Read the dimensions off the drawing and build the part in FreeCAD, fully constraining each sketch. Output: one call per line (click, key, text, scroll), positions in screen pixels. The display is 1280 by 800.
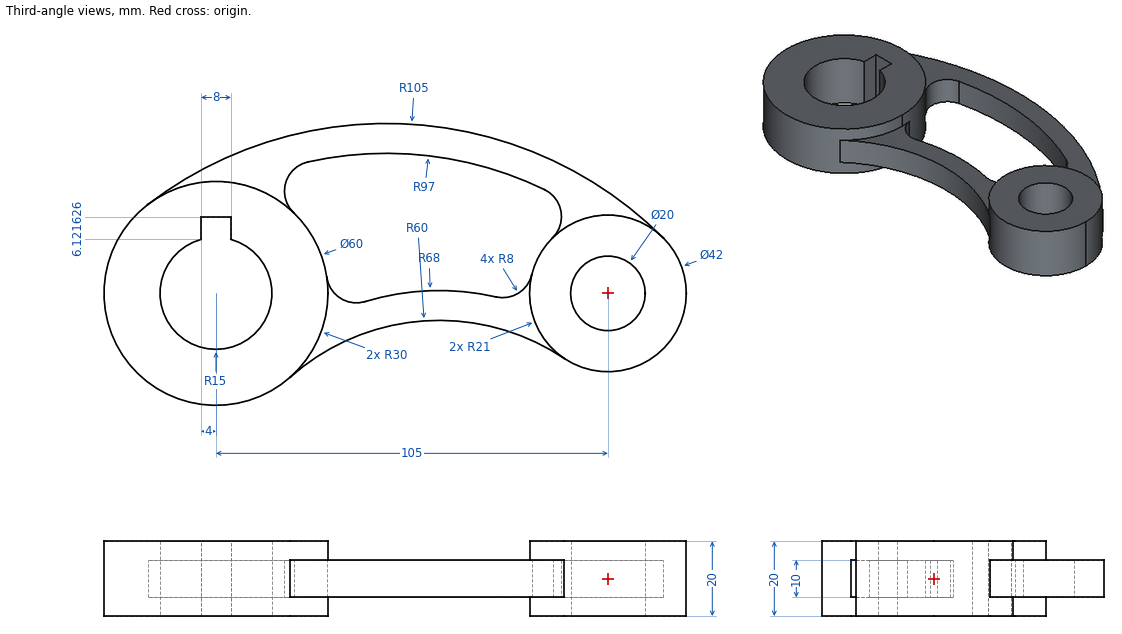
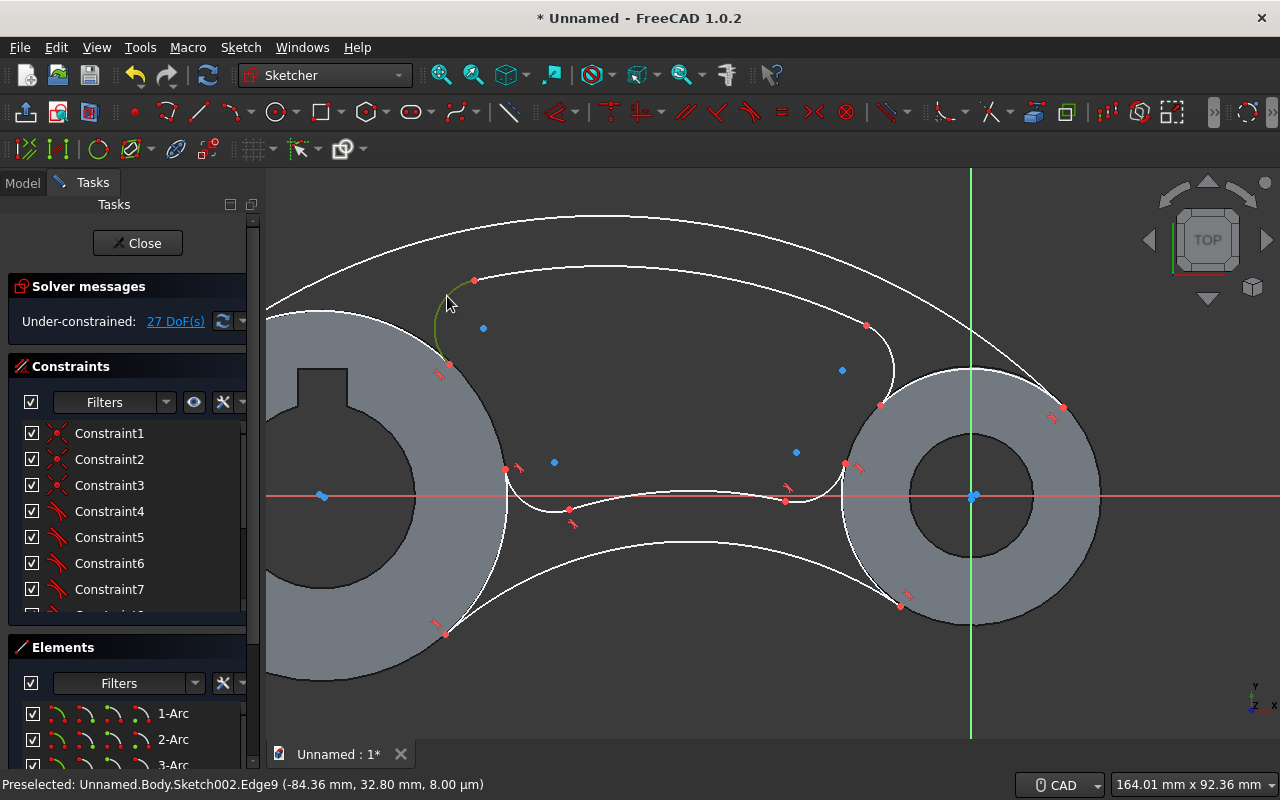
click(753, 284)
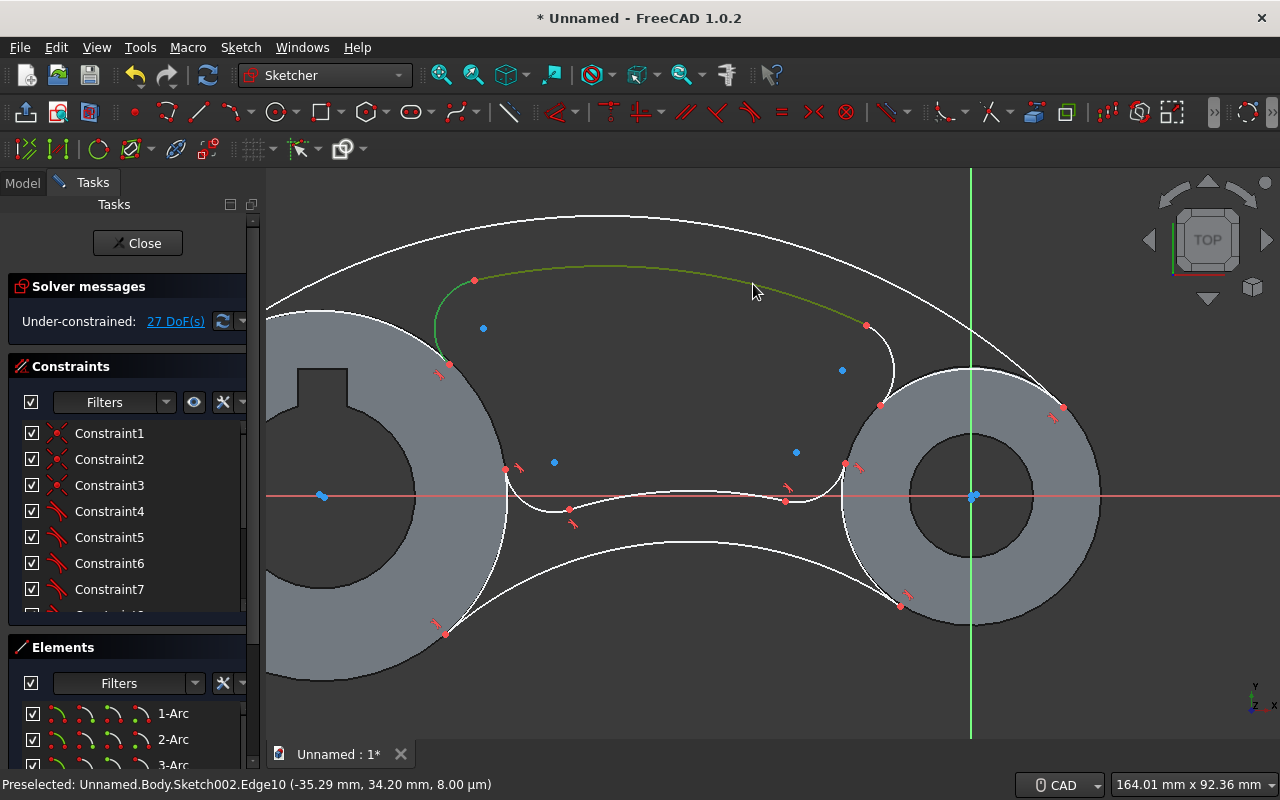
key(t)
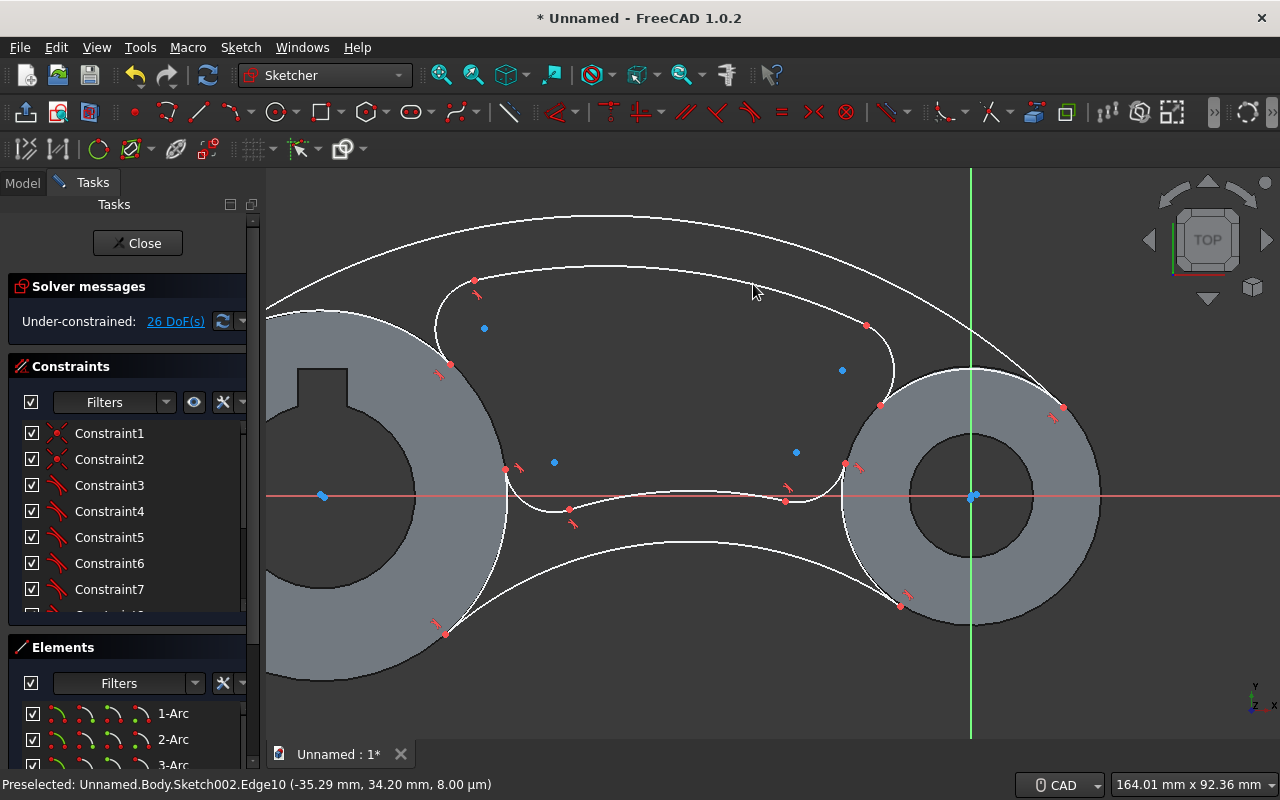
click(753, 284)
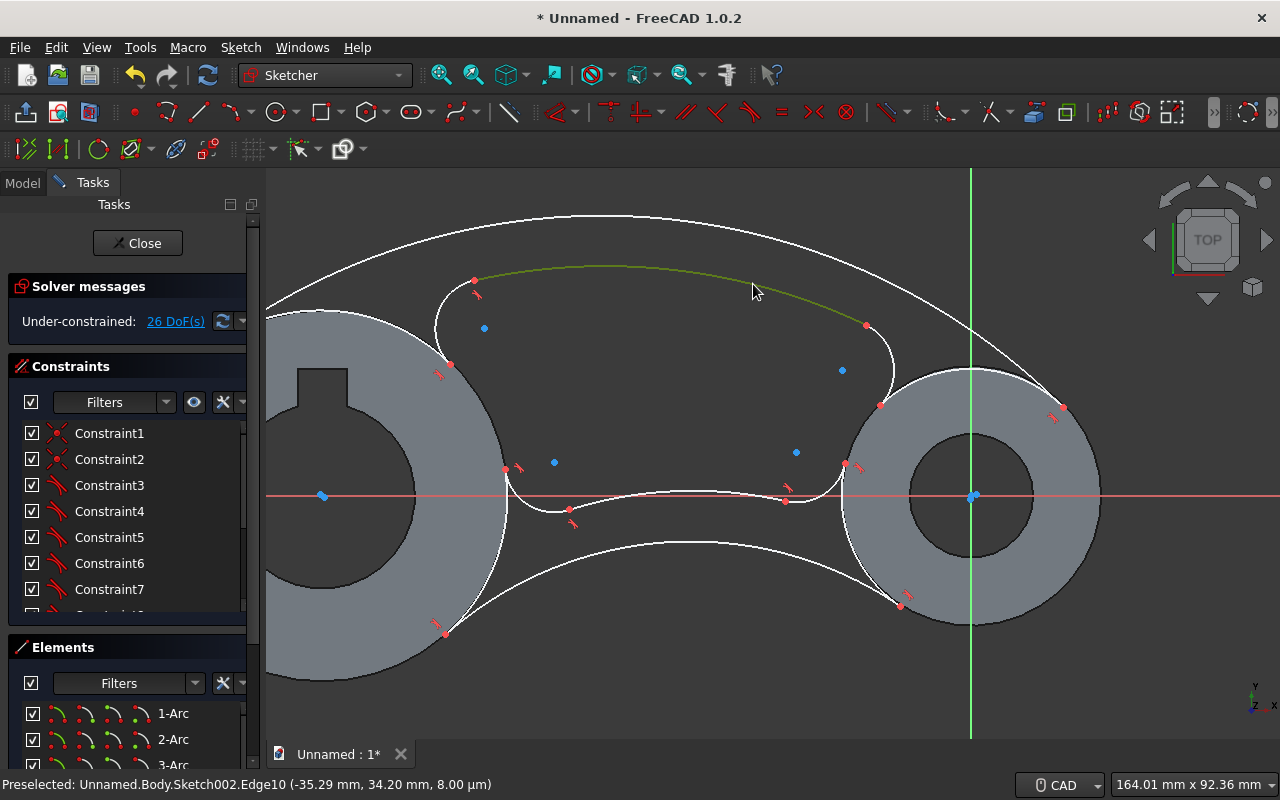
scroll(893, 381, up, 2)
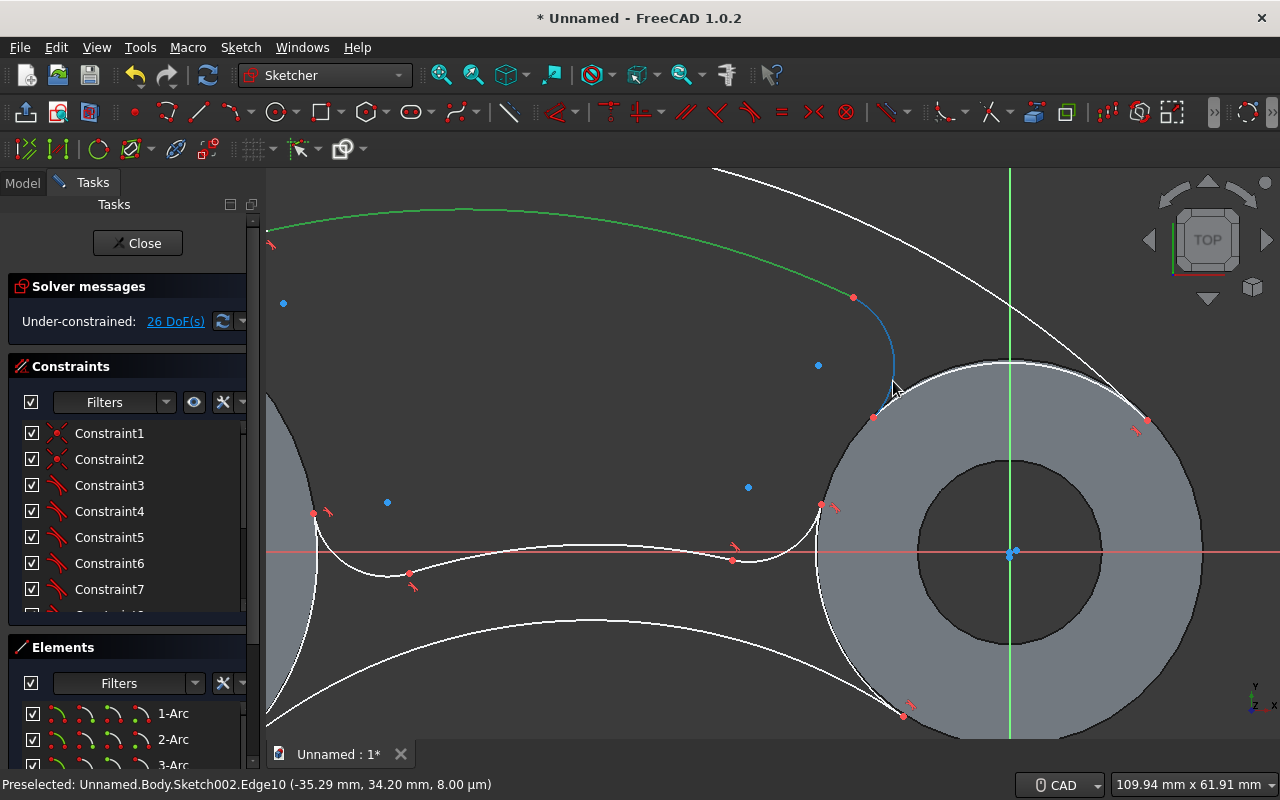
click(893, 381)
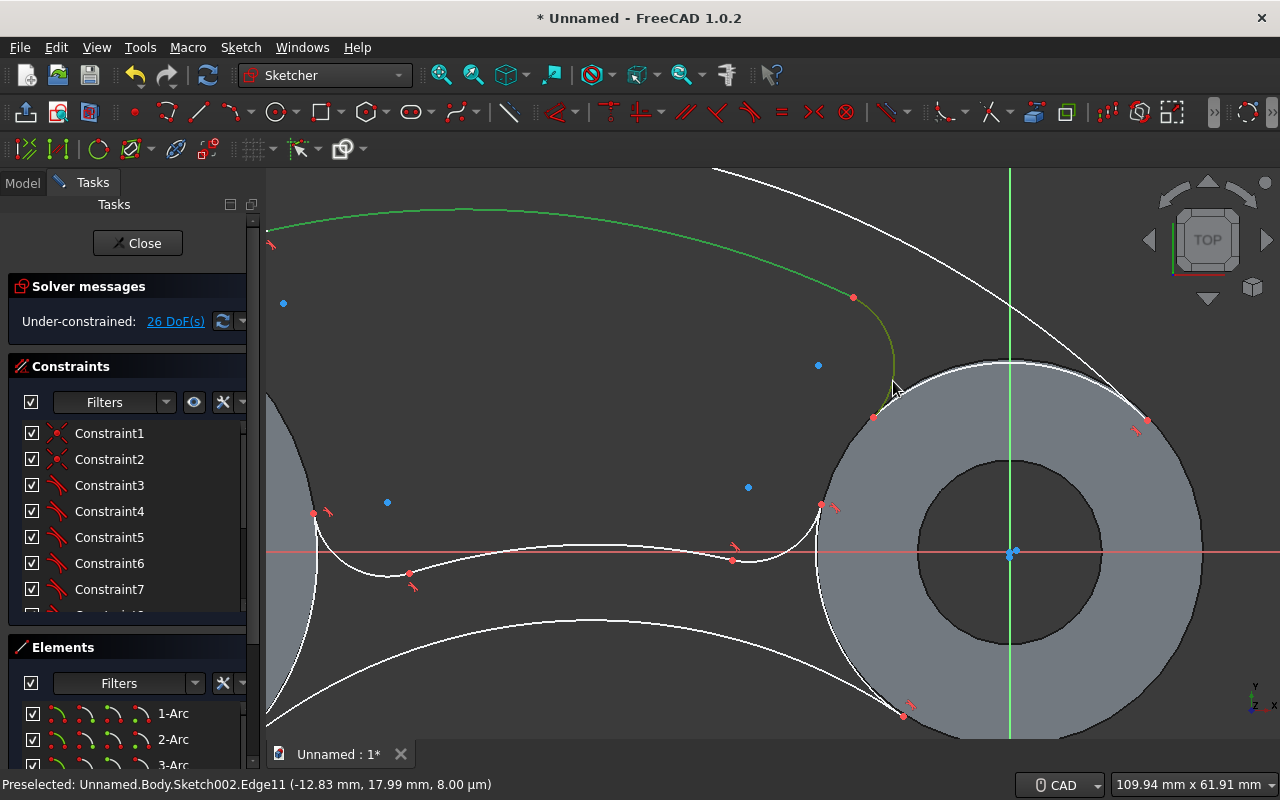
key(t)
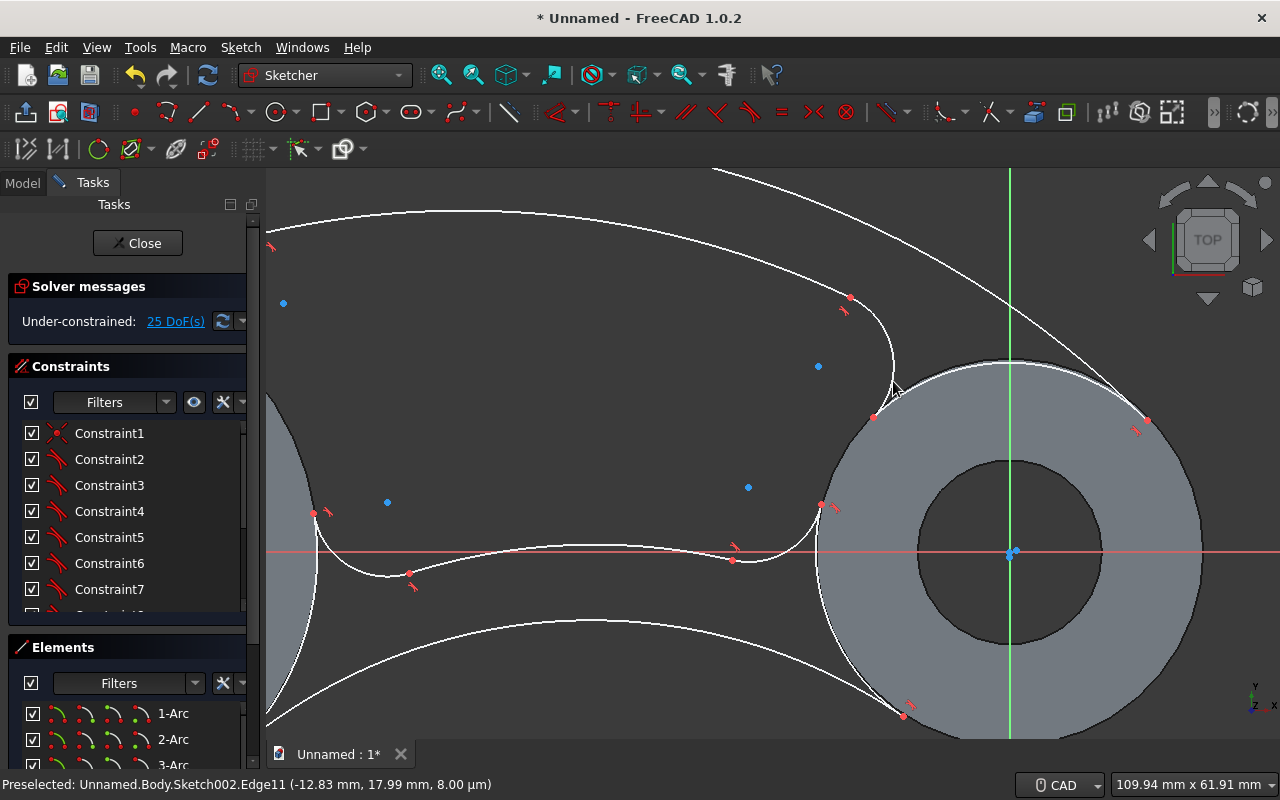
click(892, 380)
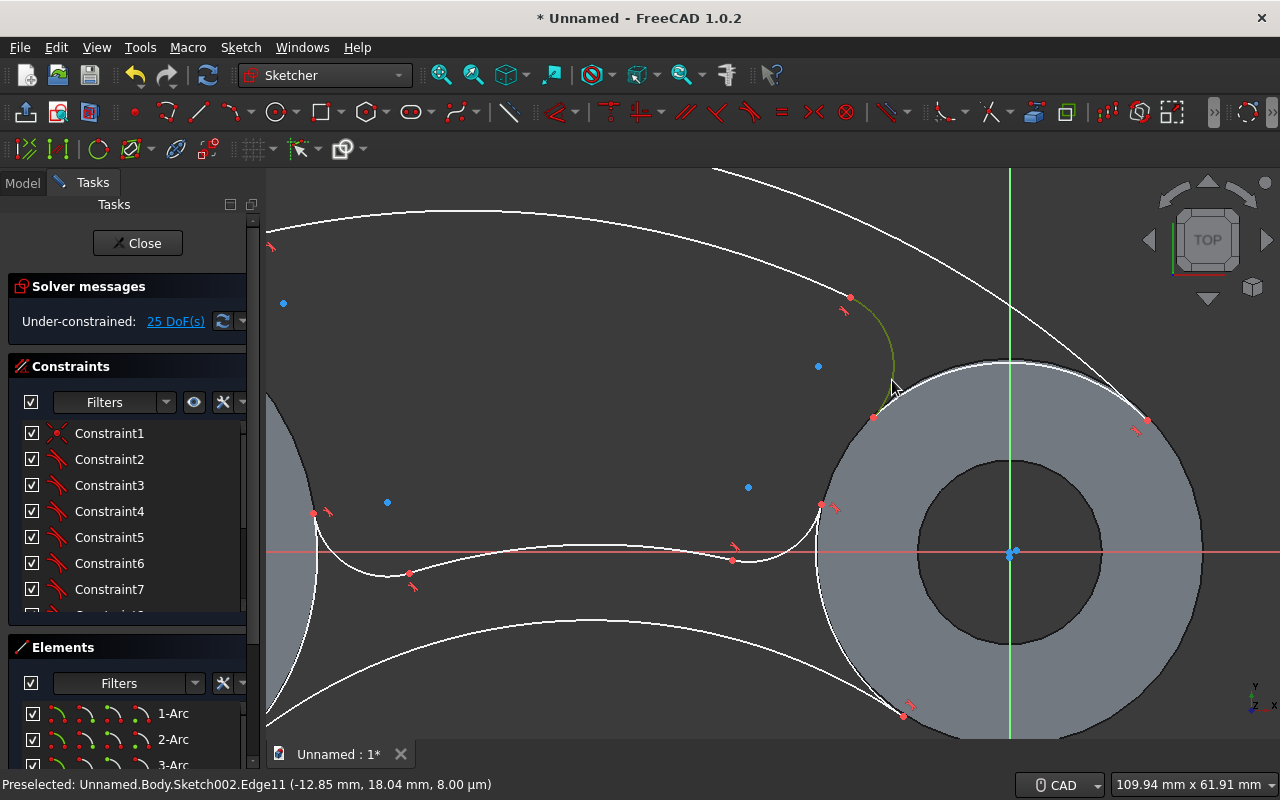
click(1070, 373)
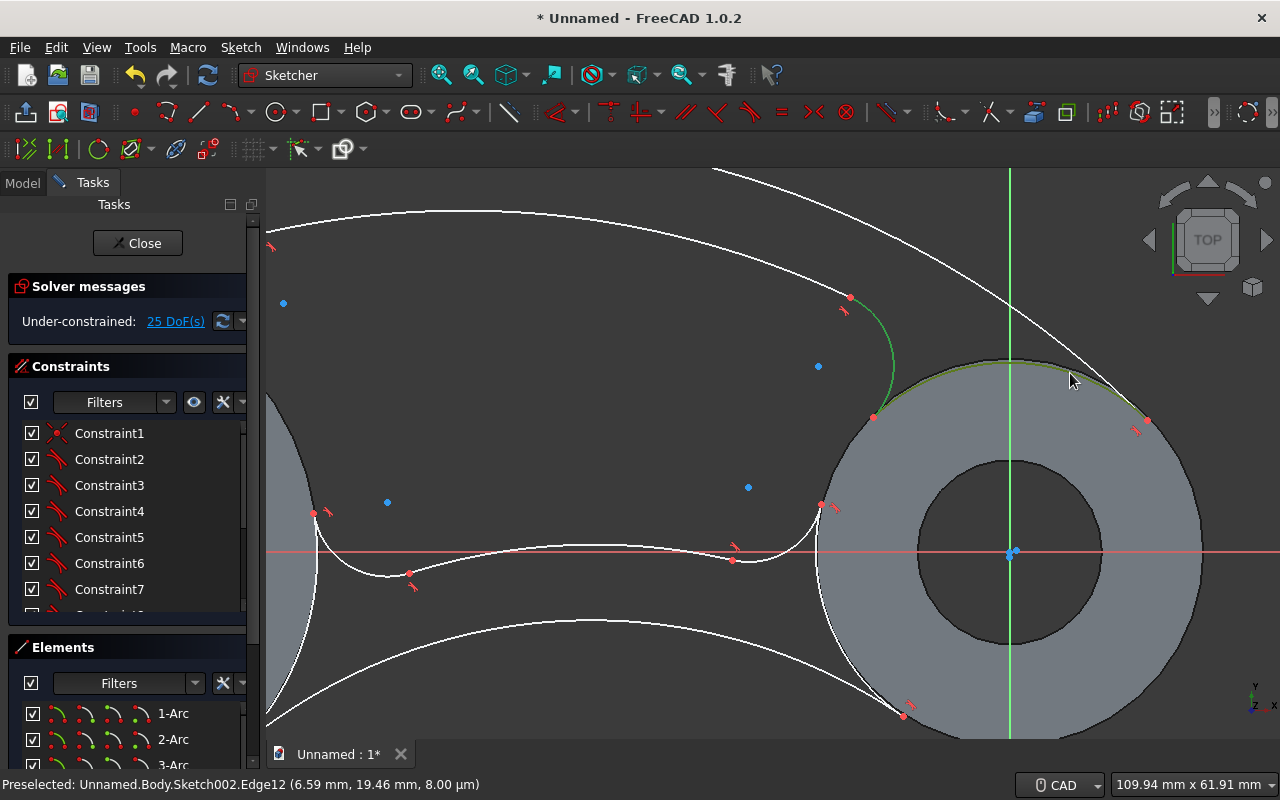
key(t)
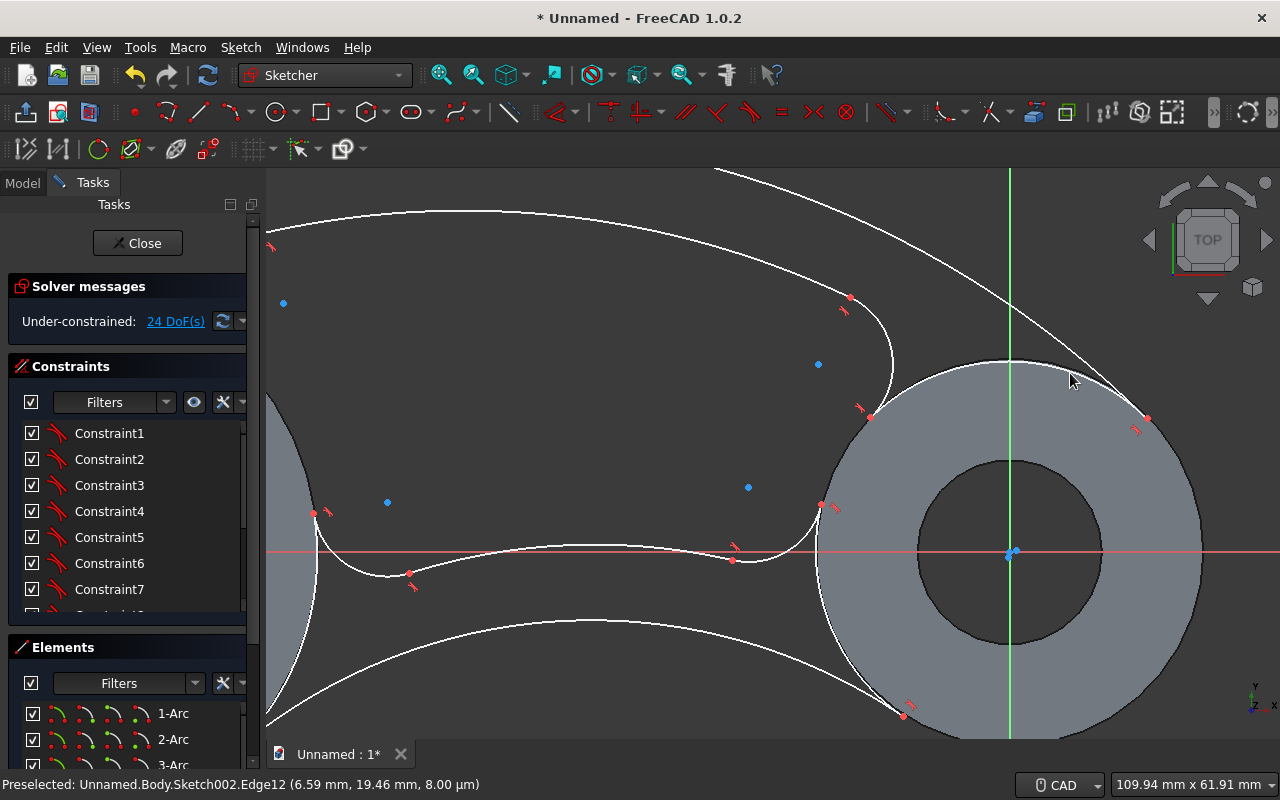
click(505, 551)